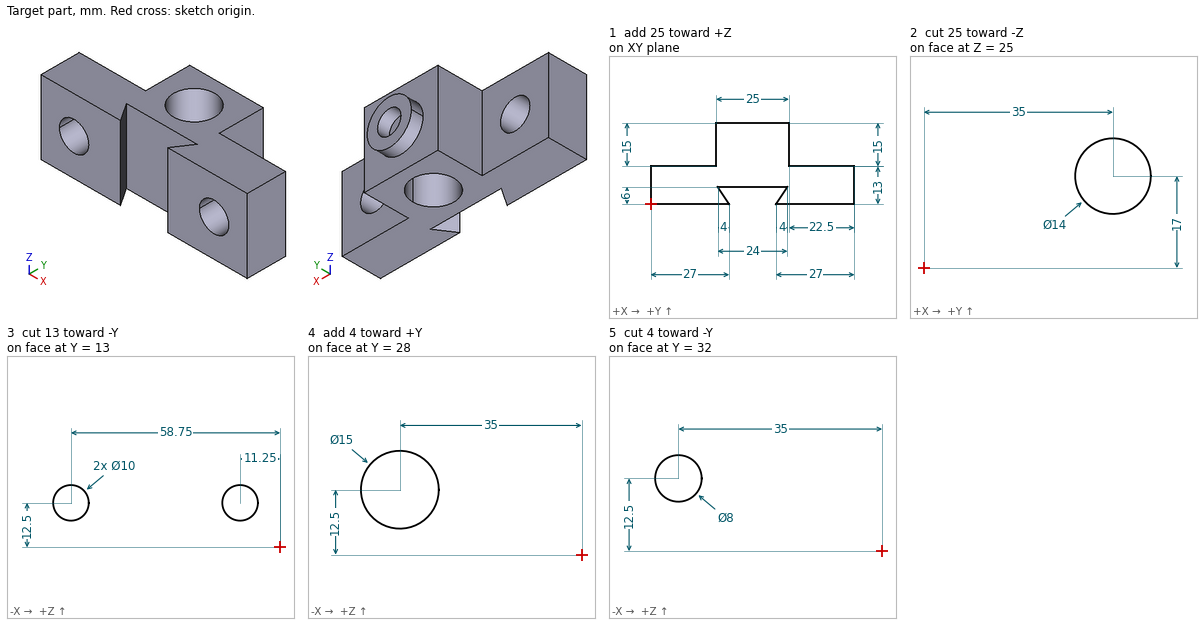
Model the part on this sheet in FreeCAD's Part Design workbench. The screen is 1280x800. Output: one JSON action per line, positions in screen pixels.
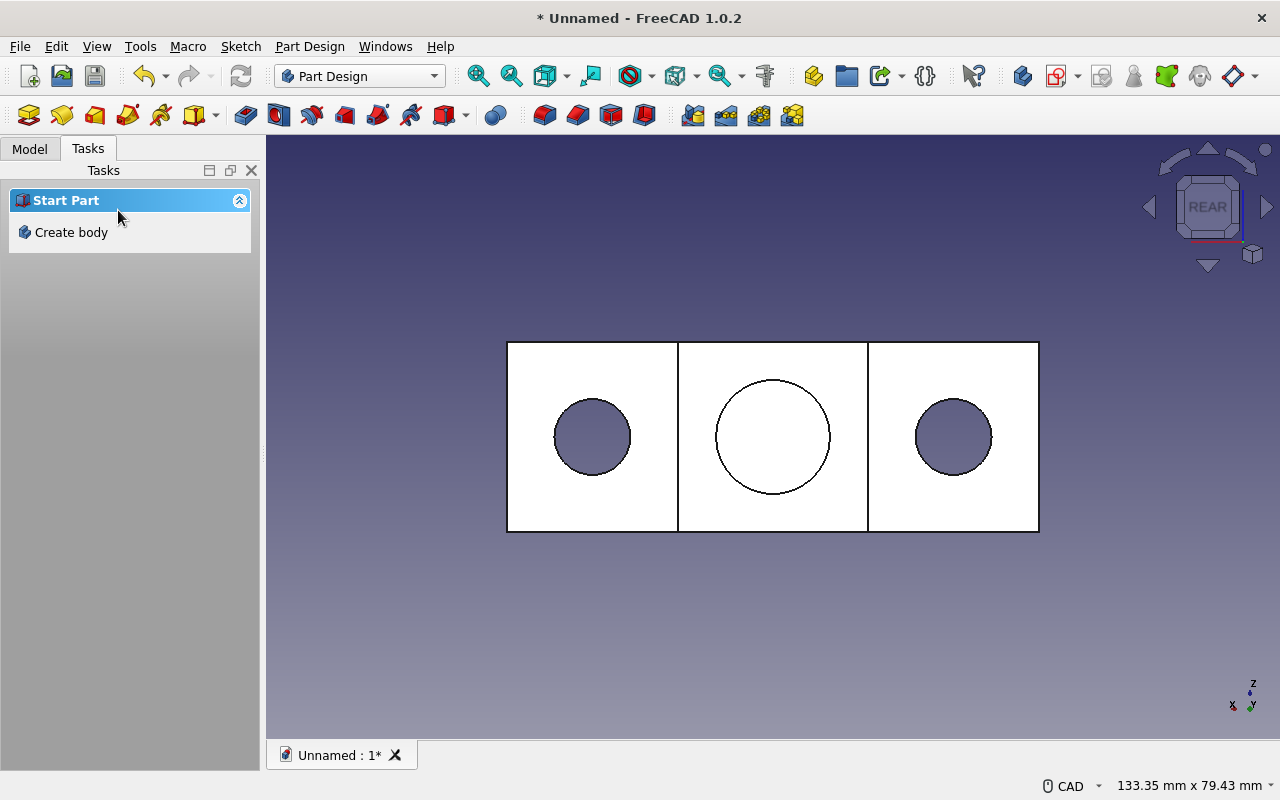
{"action": "left_click", "coordinate": [773, 436]}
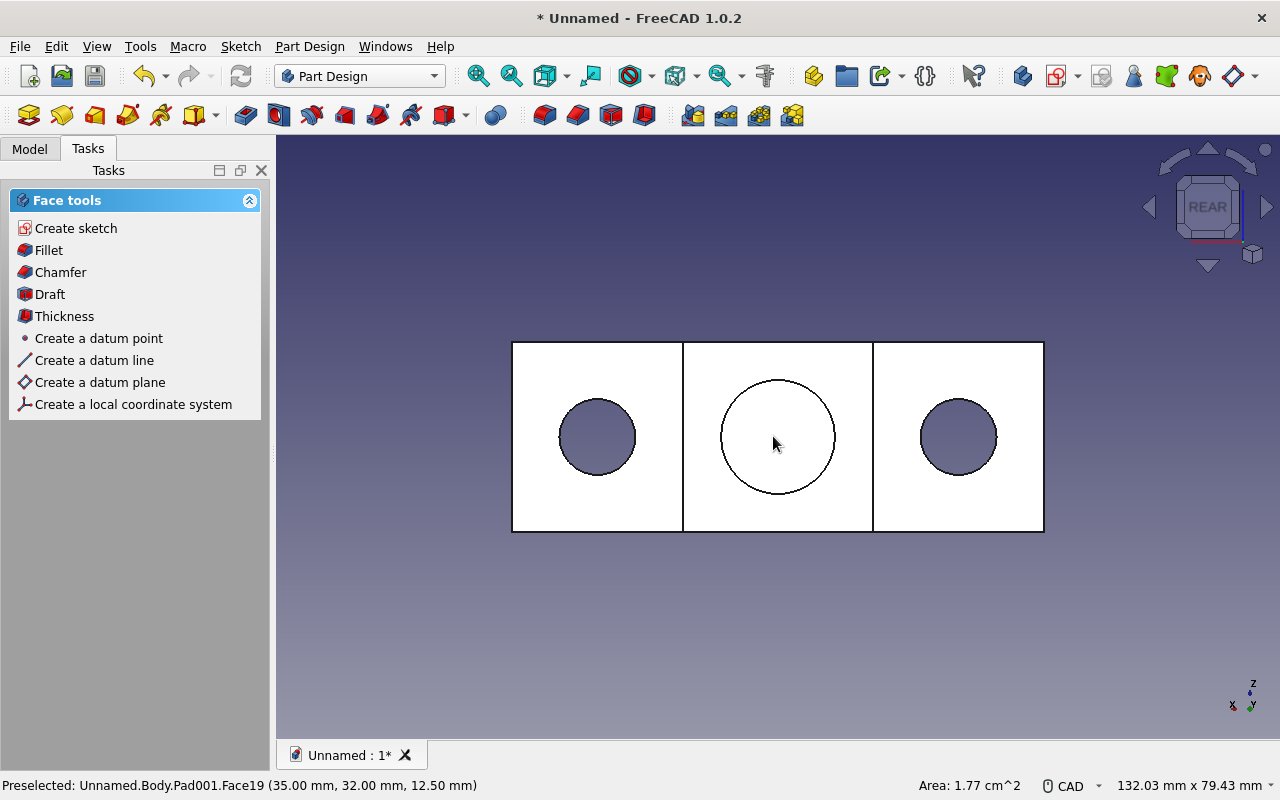
{"action": "left_click", "coordinate": [1056, 76]}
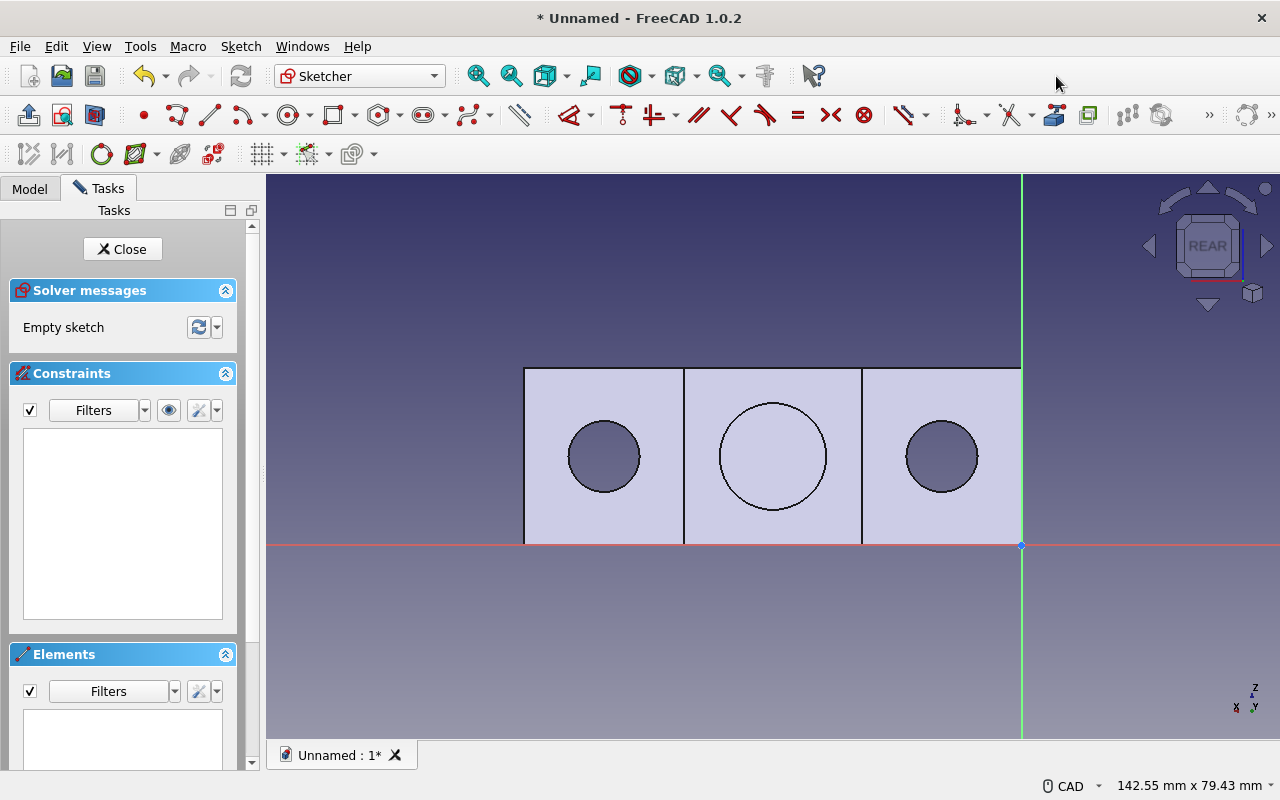
{"action": "scroll", "coordinate": [787, 457], "scroll_direction": "up", "scroll_amount": 9}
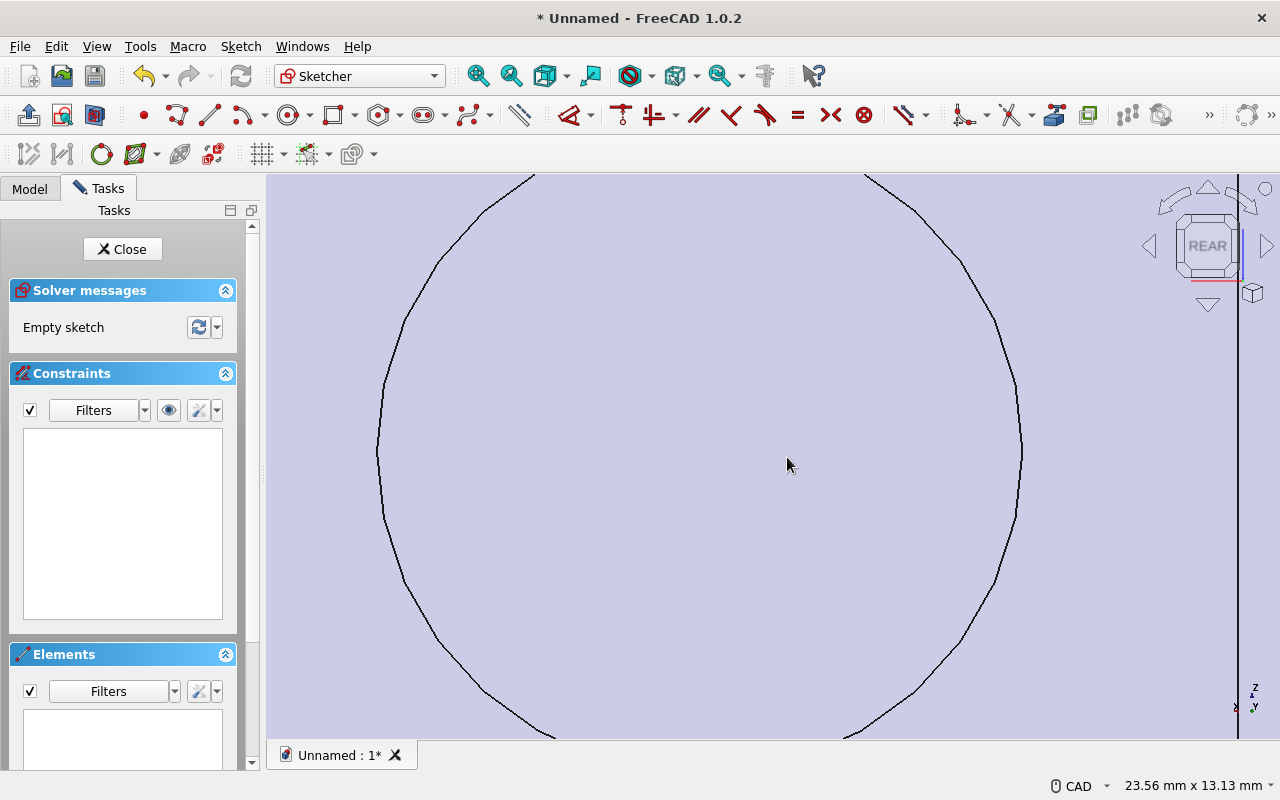
{"action": "left_click", "coordinate": [288, 116]}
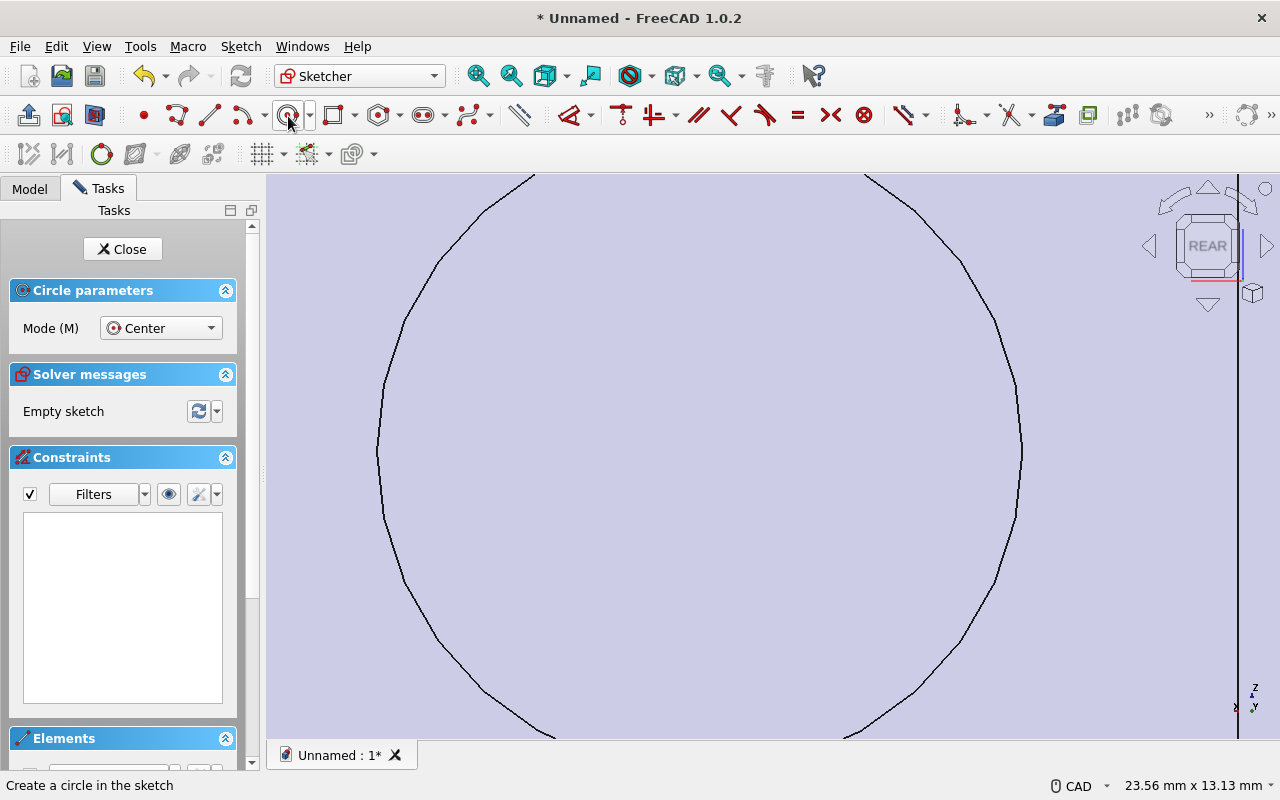
{"action": "left_click", "coordinate": [700, 451]}
{"action": "mouse_move", "coordinate": [821, 330]}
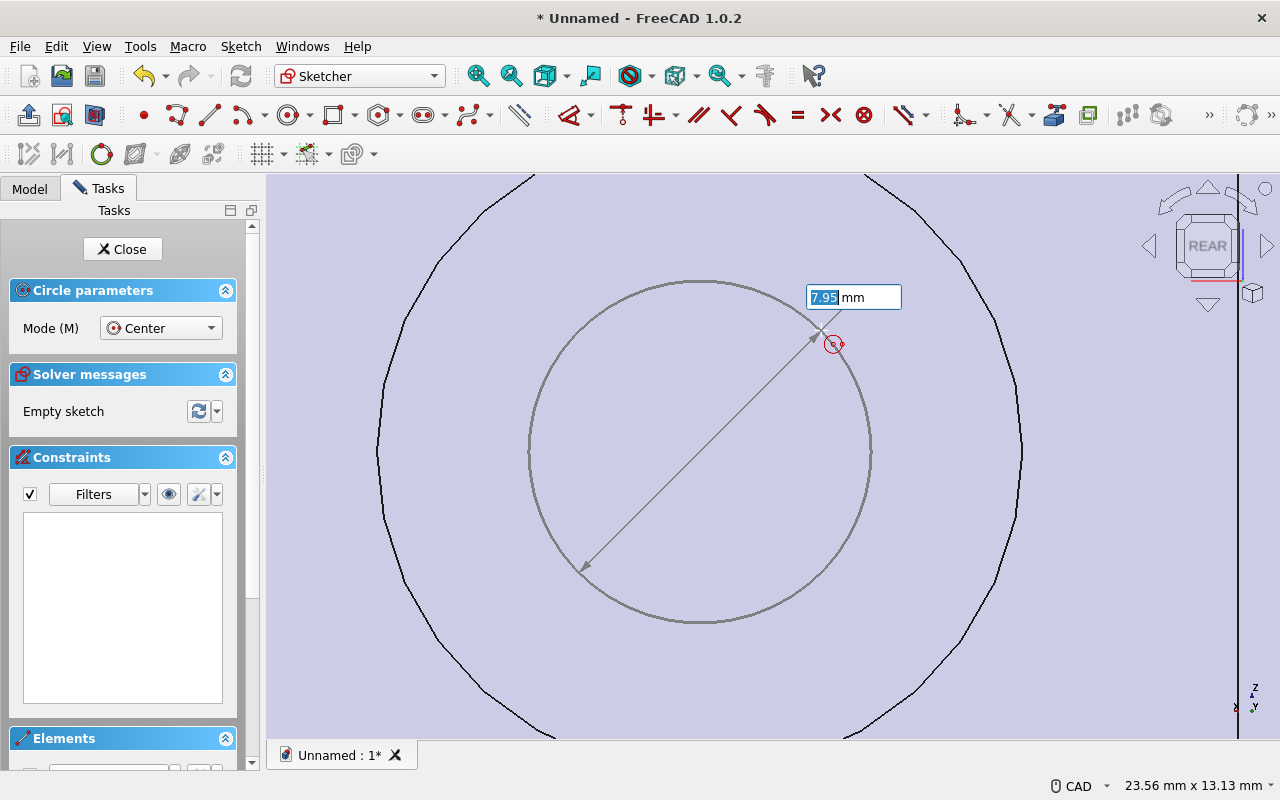
{"action": "type", "text": "8"}
{"action": "key", "text": "Return"}
{"action": "key", "text": "Escape"}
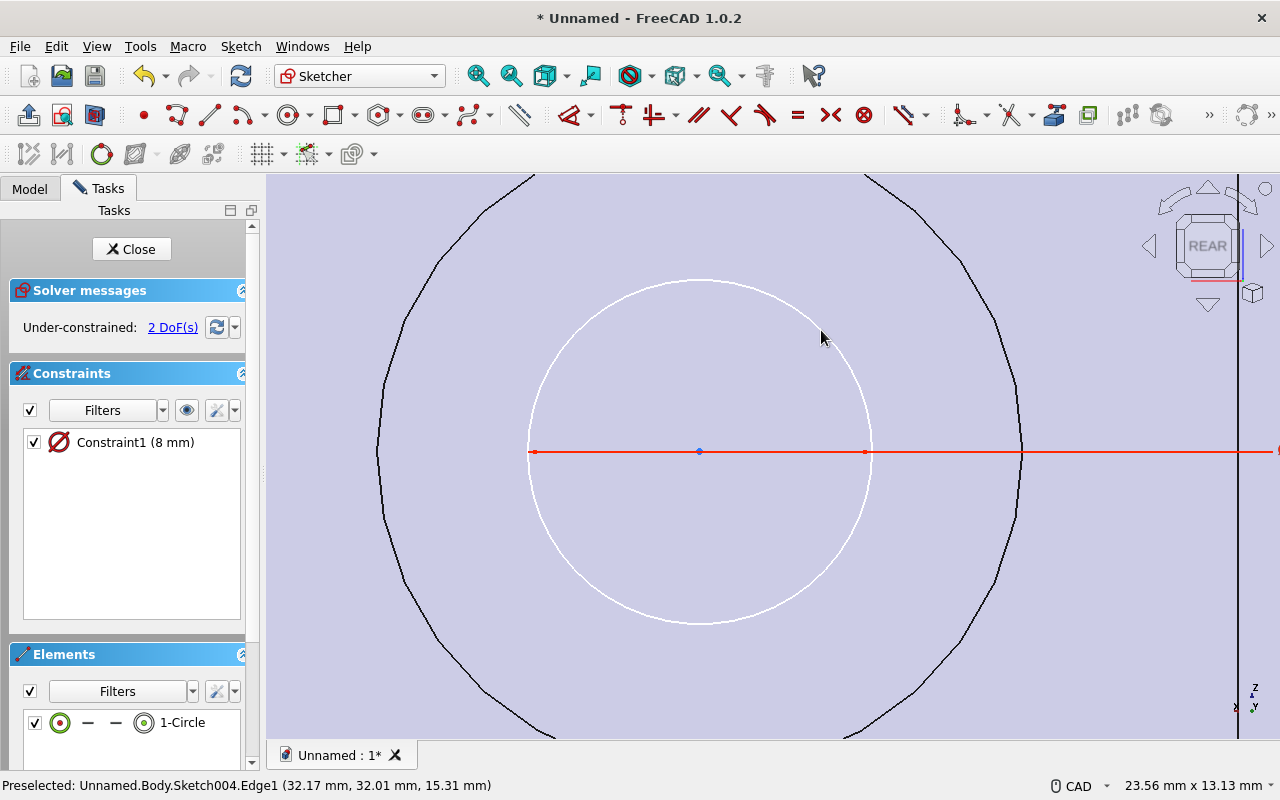
{"action": "left_click", "coordinate": [568, 116]}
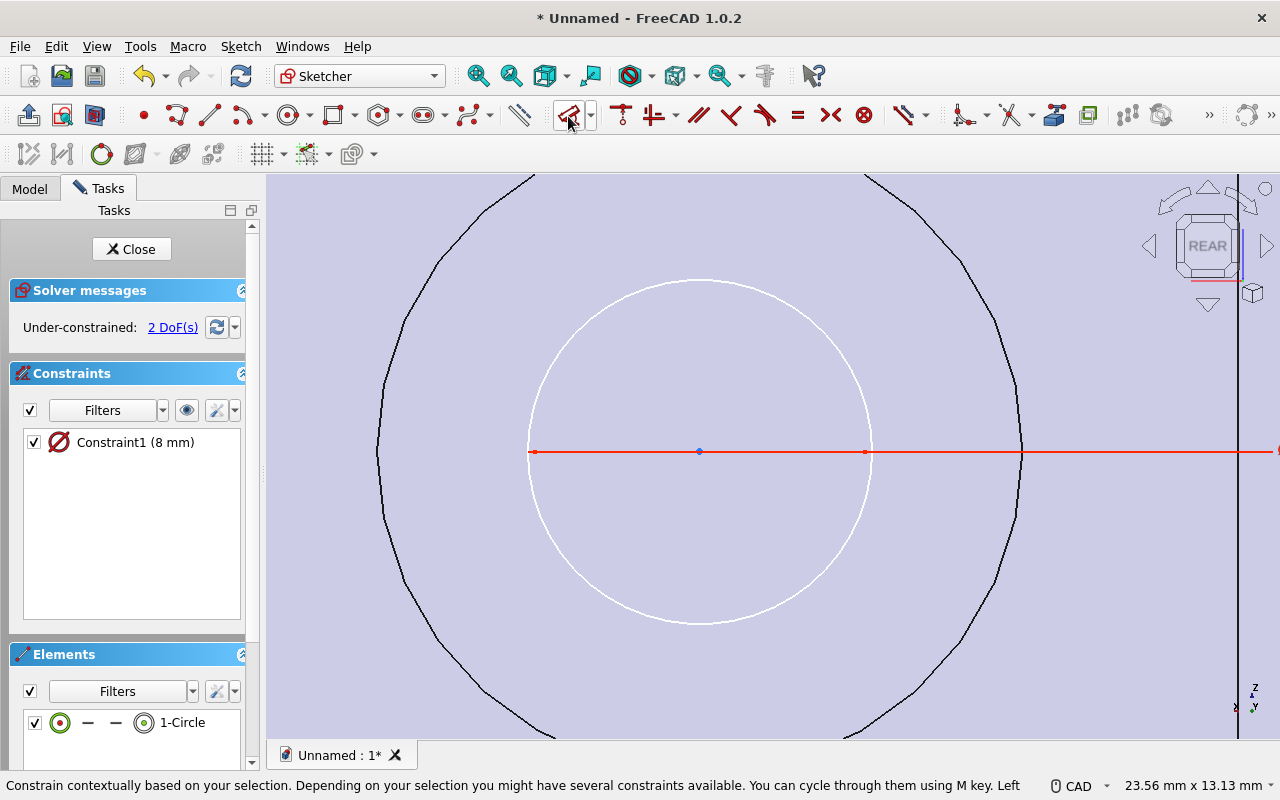
{"action": "left_click", "coordinate": [700, 452]}
{"action": "left_click", "coordinate": [908, 418]}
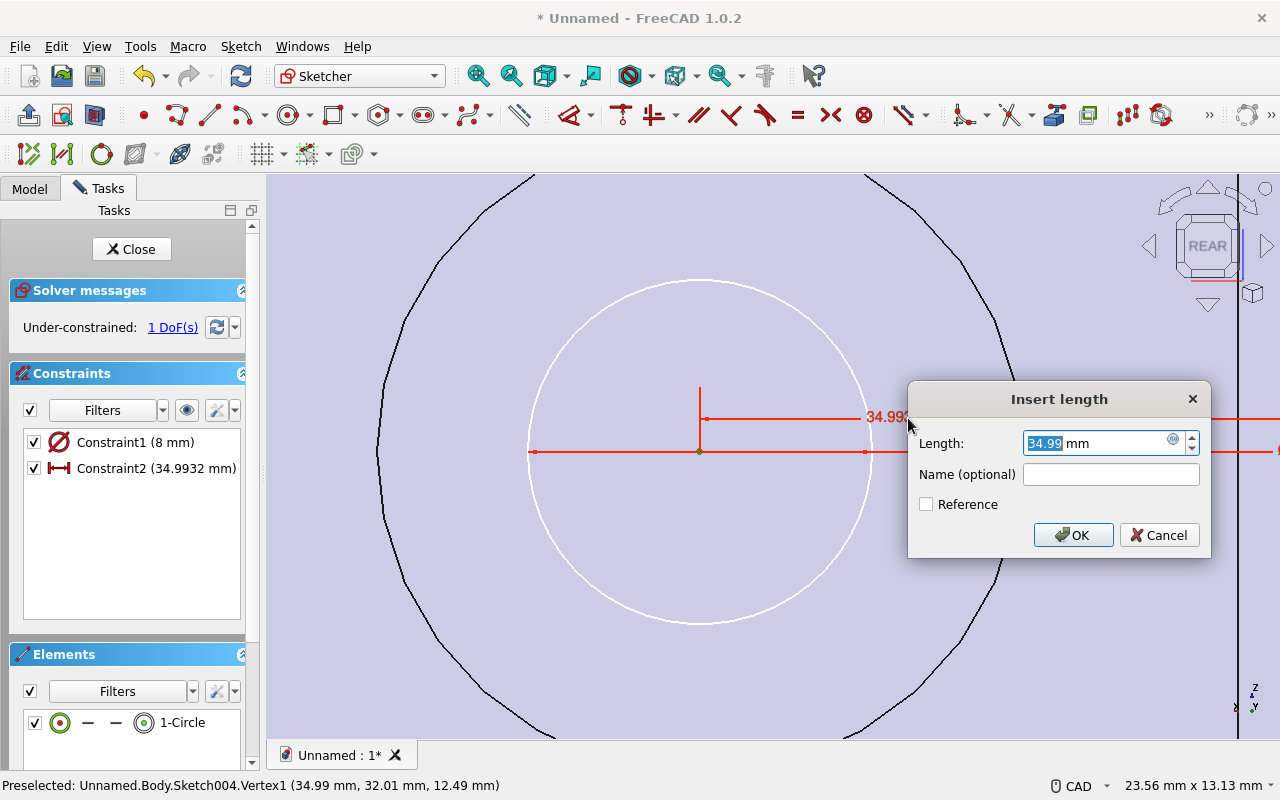
{"action": "type", "text": "35"}
{"action": "key", "text": "Return"}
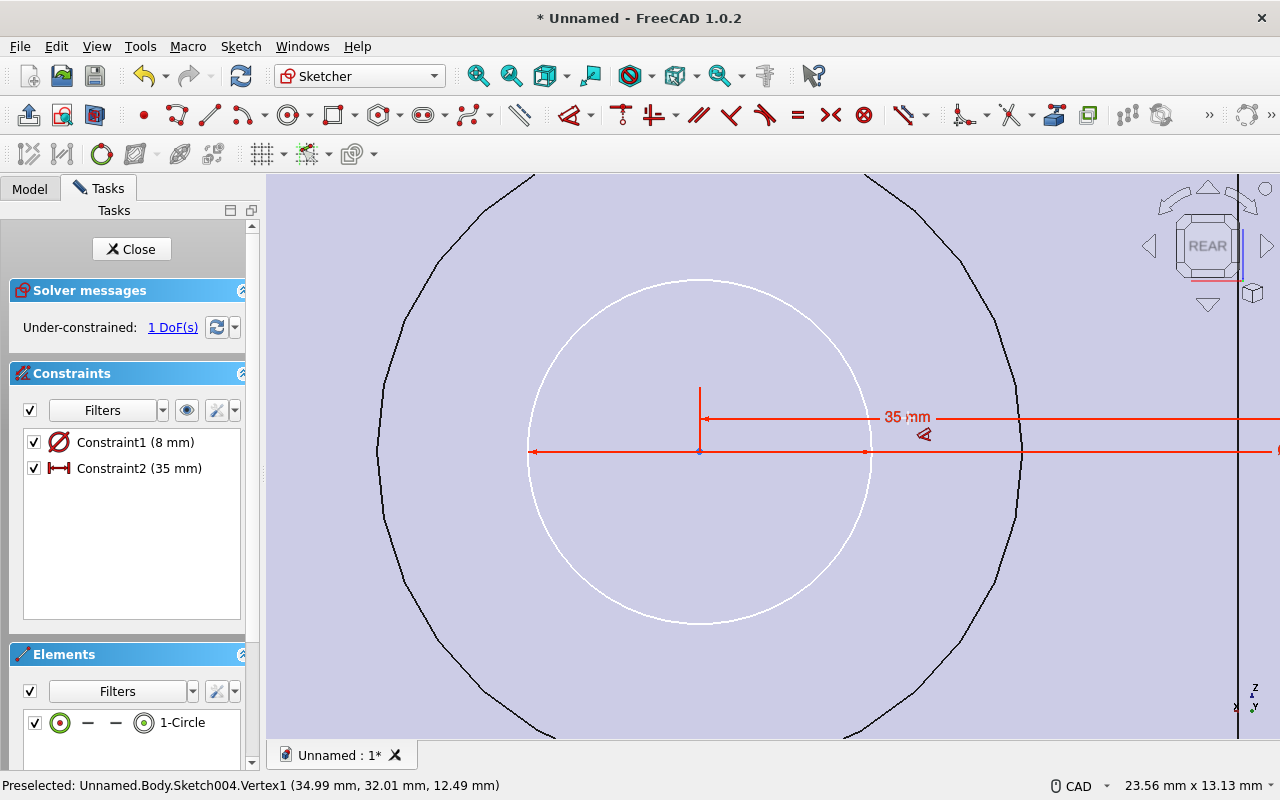
{"action": "left_click", "coordinate": [700, 452]}
{"action": "left_click", "coordinate": [666, 581]}